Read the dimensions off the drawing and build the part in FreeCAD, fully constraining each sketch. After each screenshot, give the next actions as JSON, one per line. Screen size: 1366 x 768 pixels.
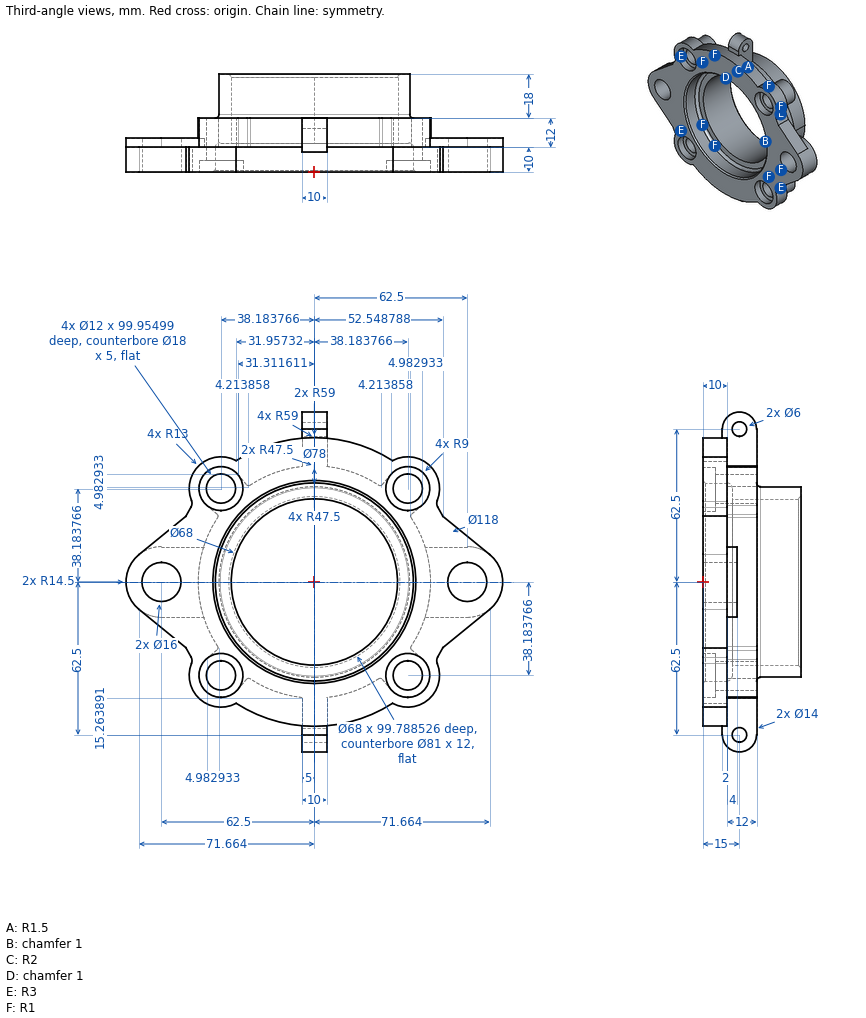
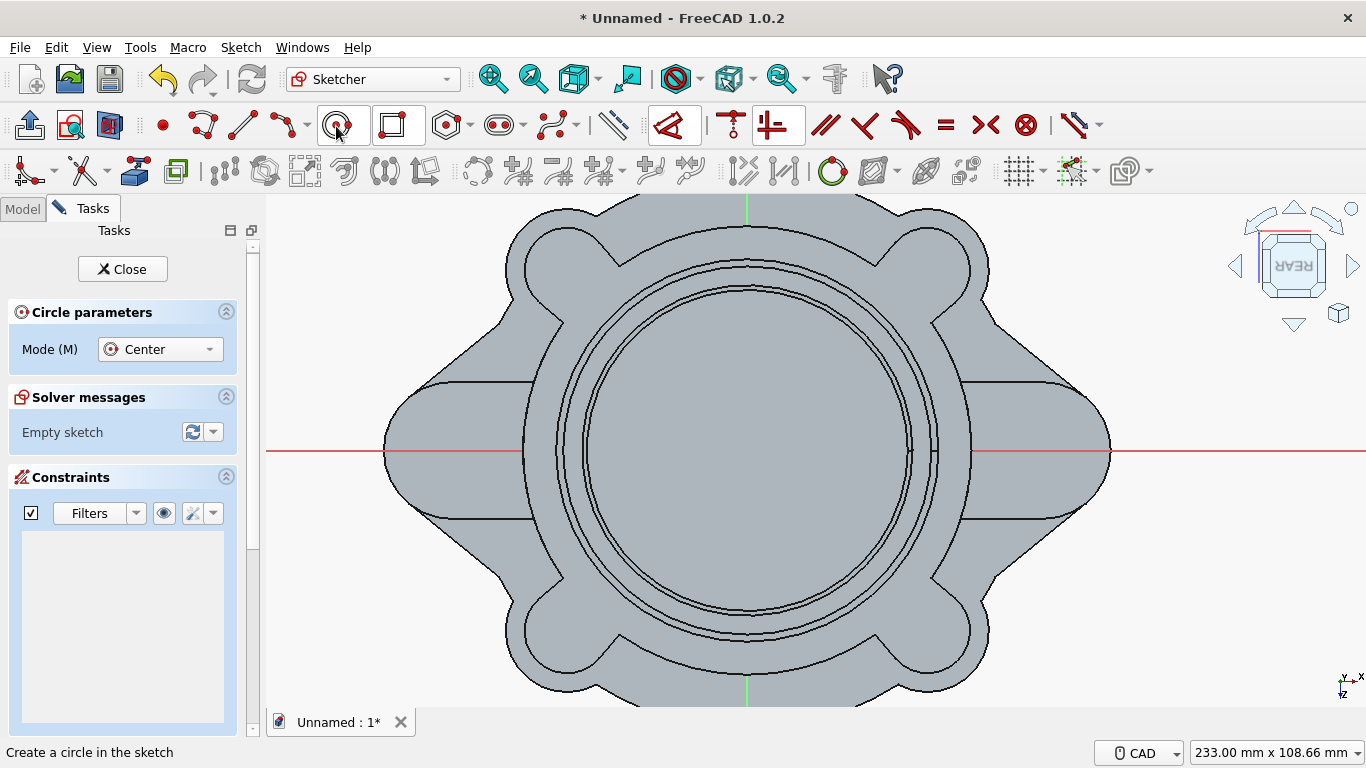
{"action": "left_click", "coordinate": [452, 450]}
{"action": "left_click", "coordinate": [479, 424]}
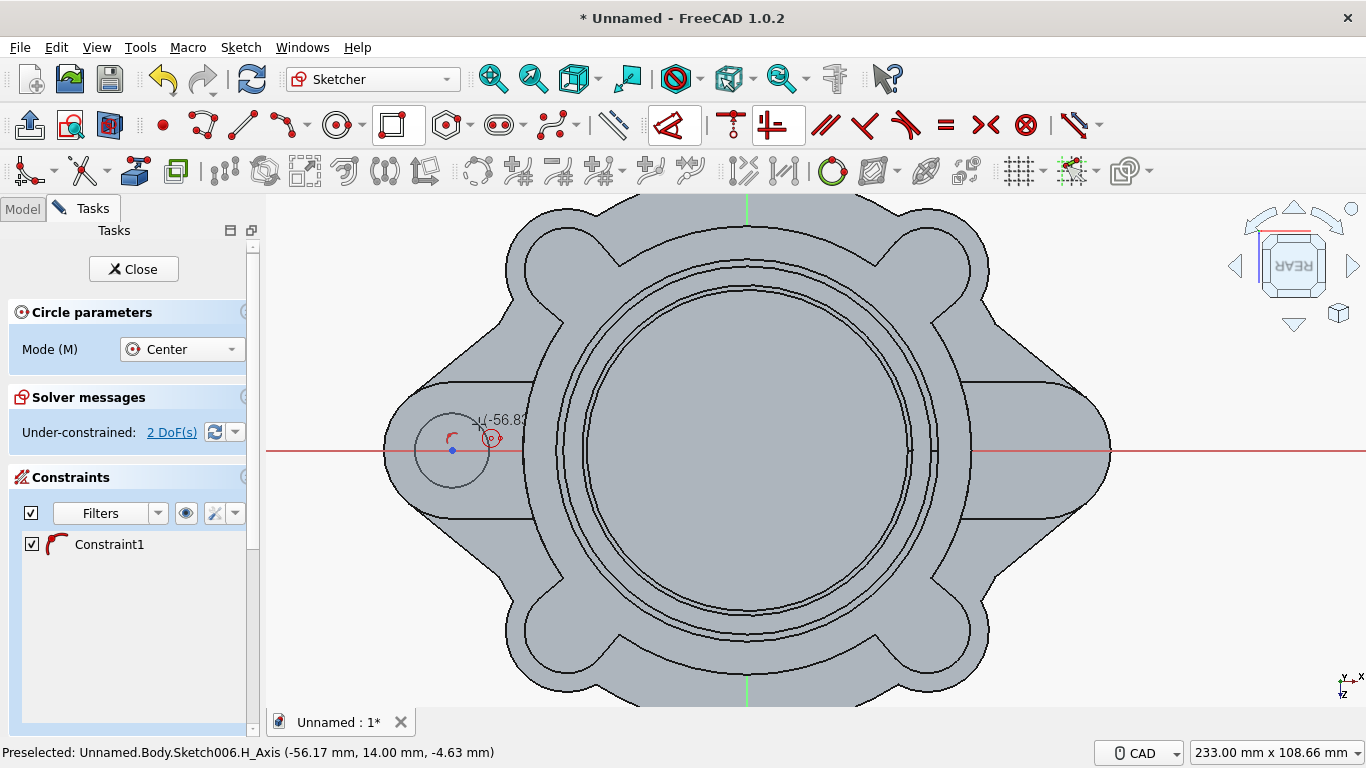
{"action": "left_click", "coordinate": [1042, 450]}
{"action": "left_click", "coordinate": [1069, 424]}
{"action": "key", "text": "Escape"}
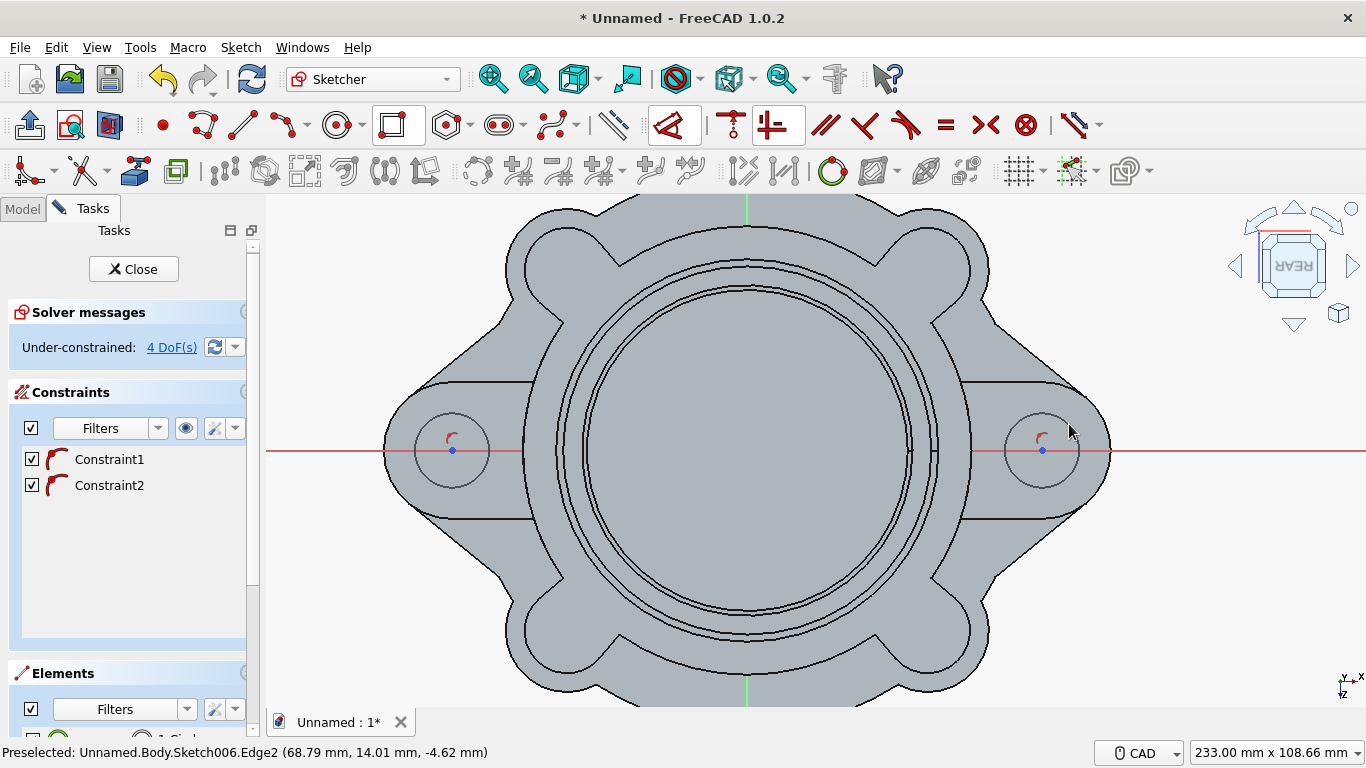
{"action": "left_click", "coordinate": [478, 424]}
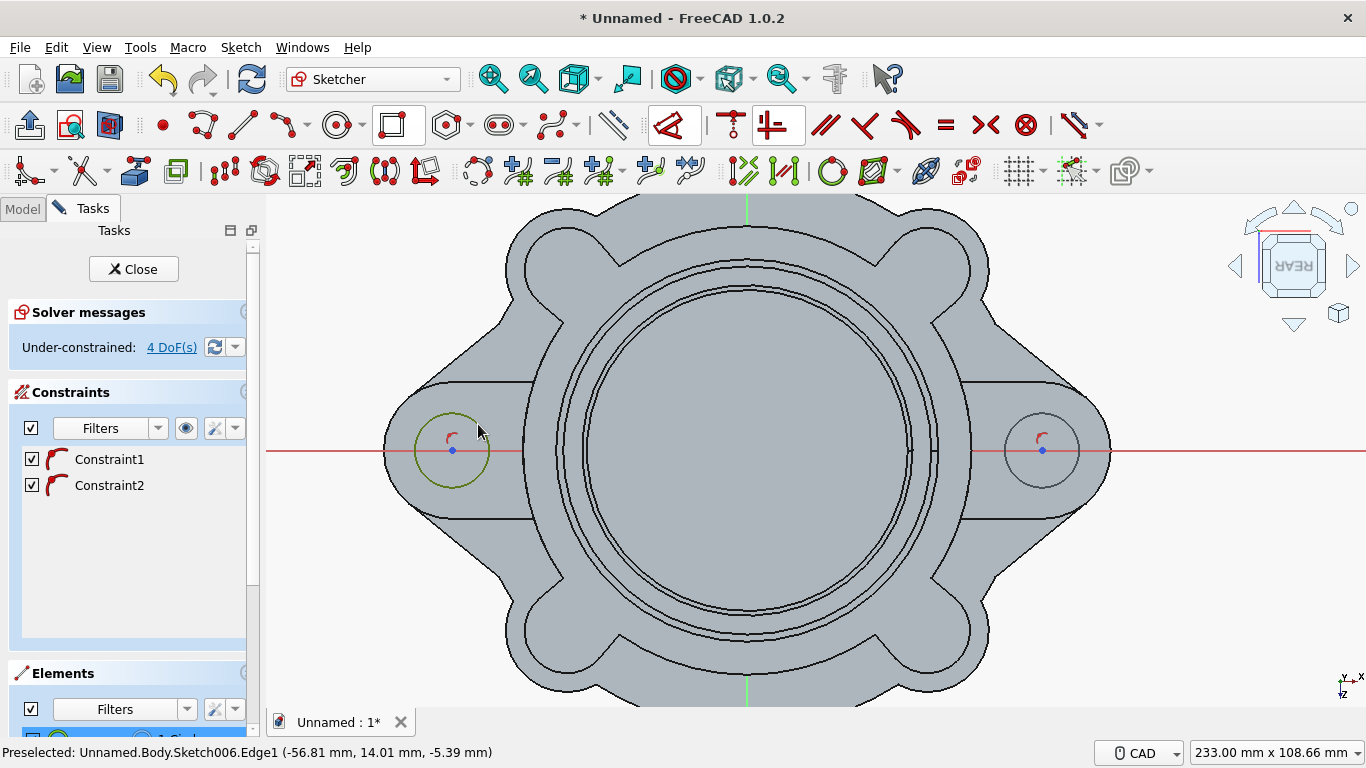
{"action": "left_click", "coordinate": [1068, 424]}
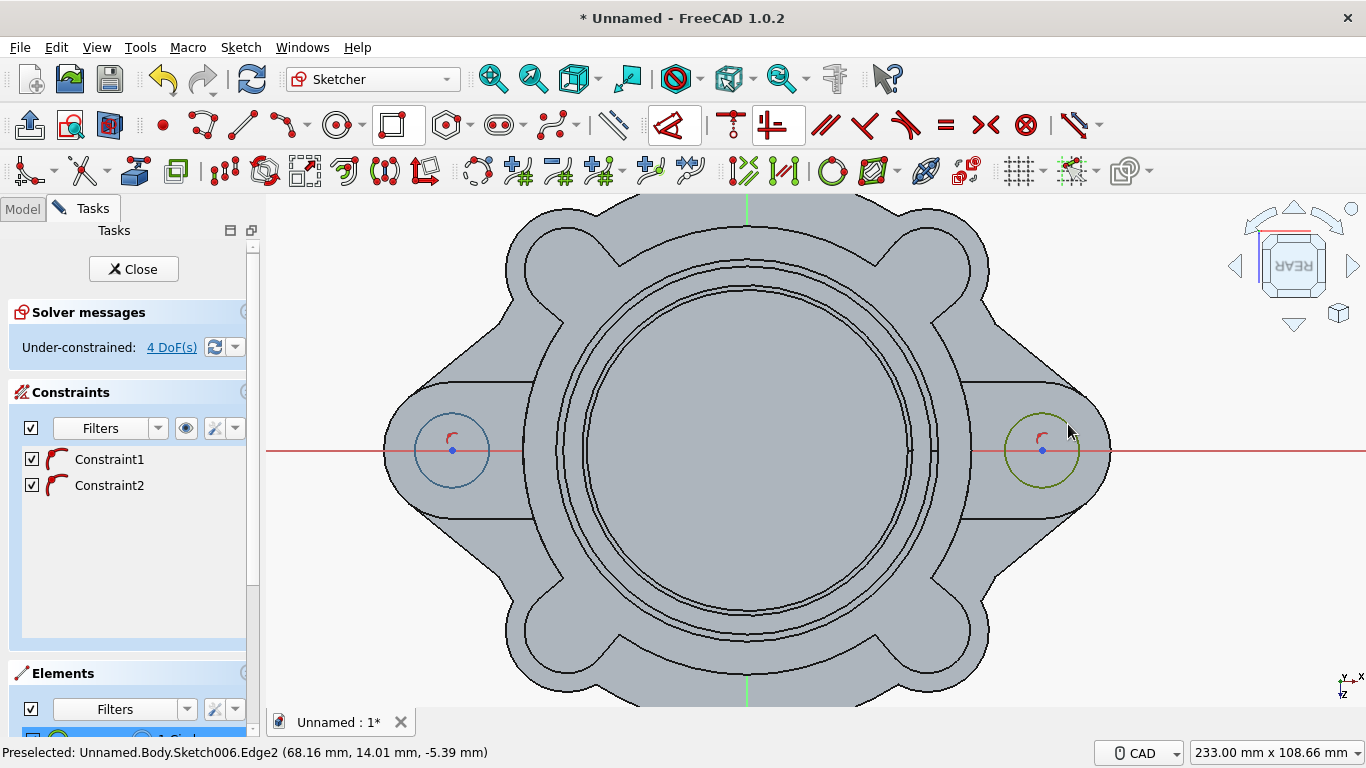
{"action": "left_click", "coordinate": [946, 126]}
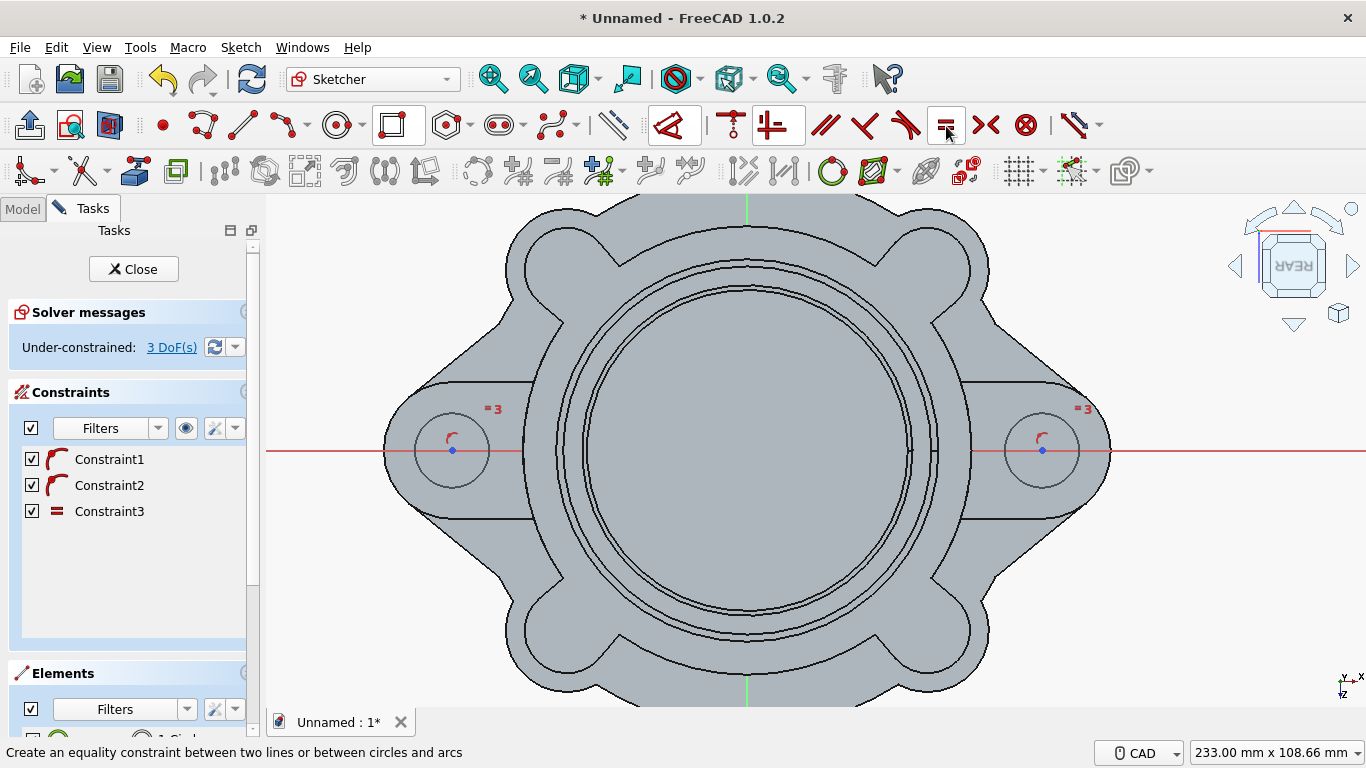
{"action": "left_click", "coordinate": [478, 424]}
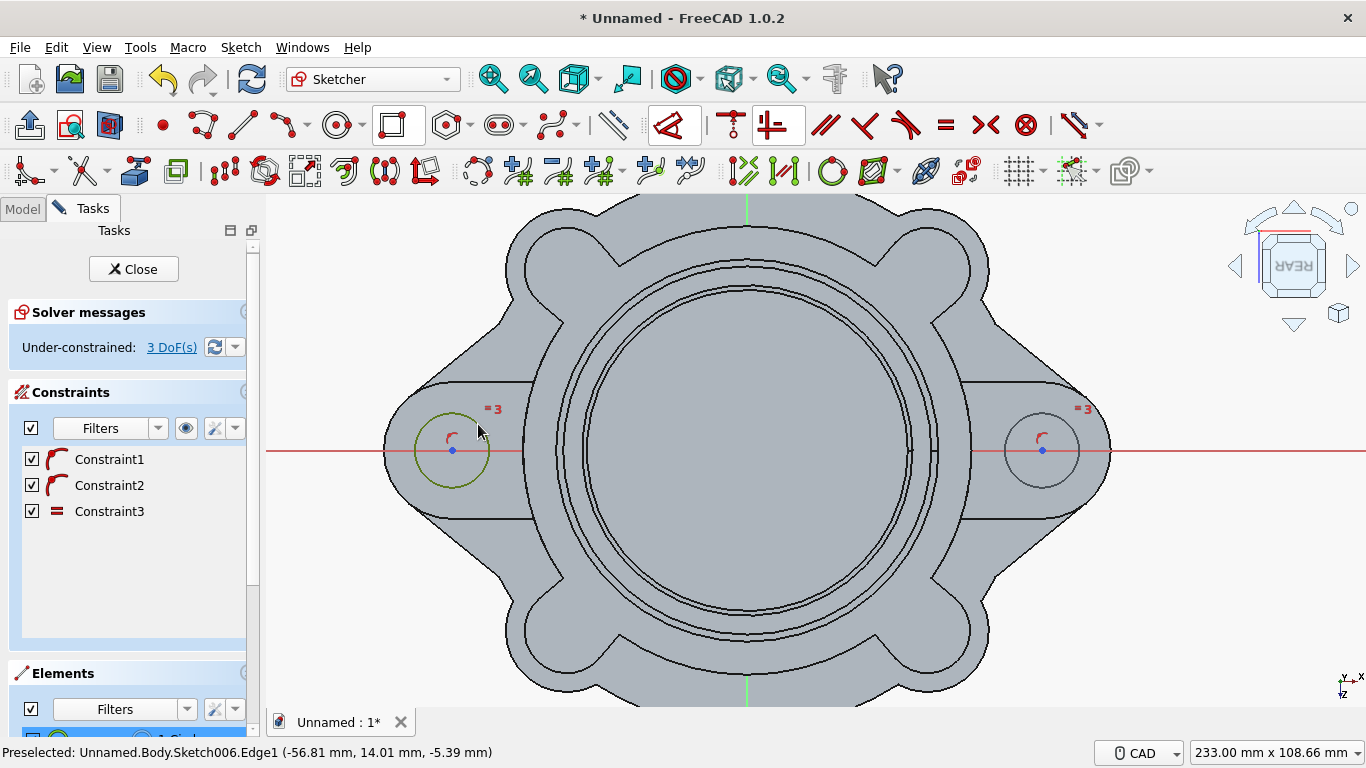
{"action": "left_click", "coordinate": [696, 126]}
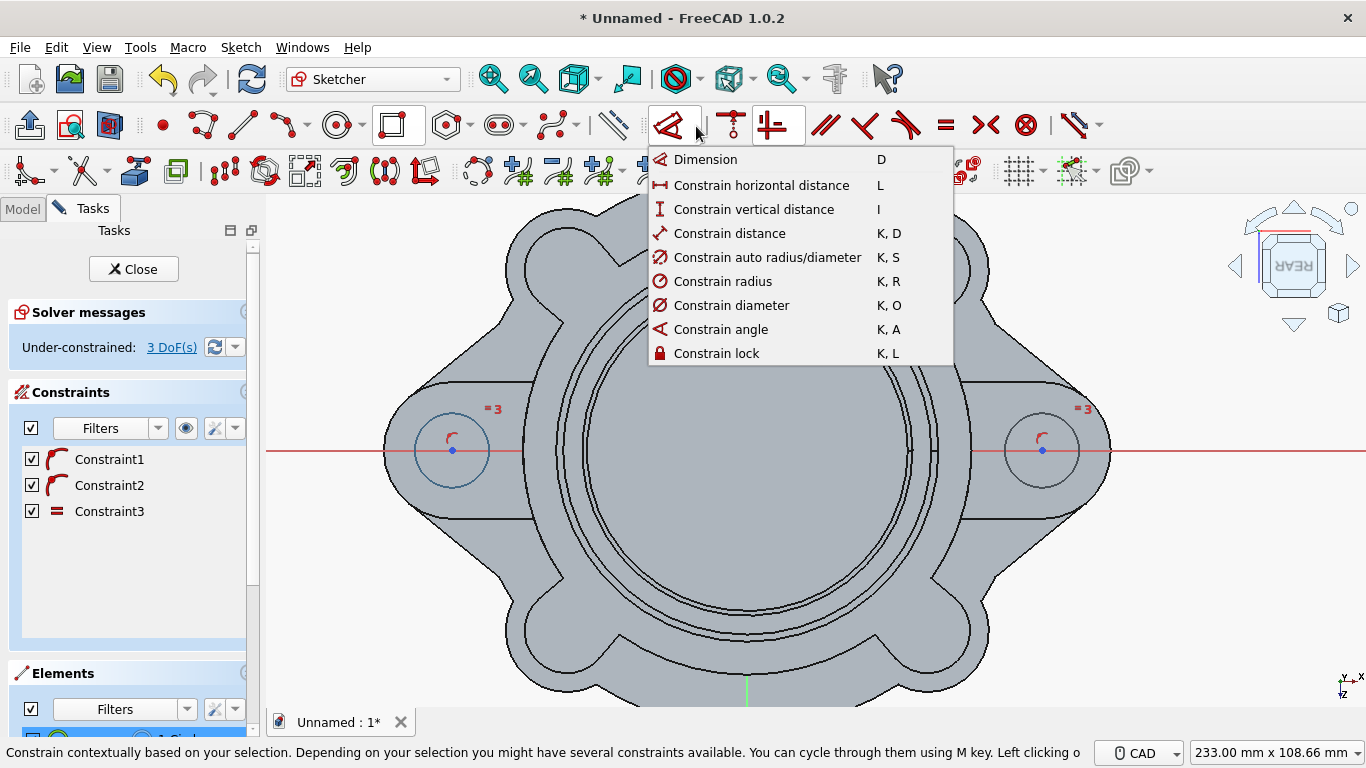
{"action": "left_click", "coordinate": [801, 305]}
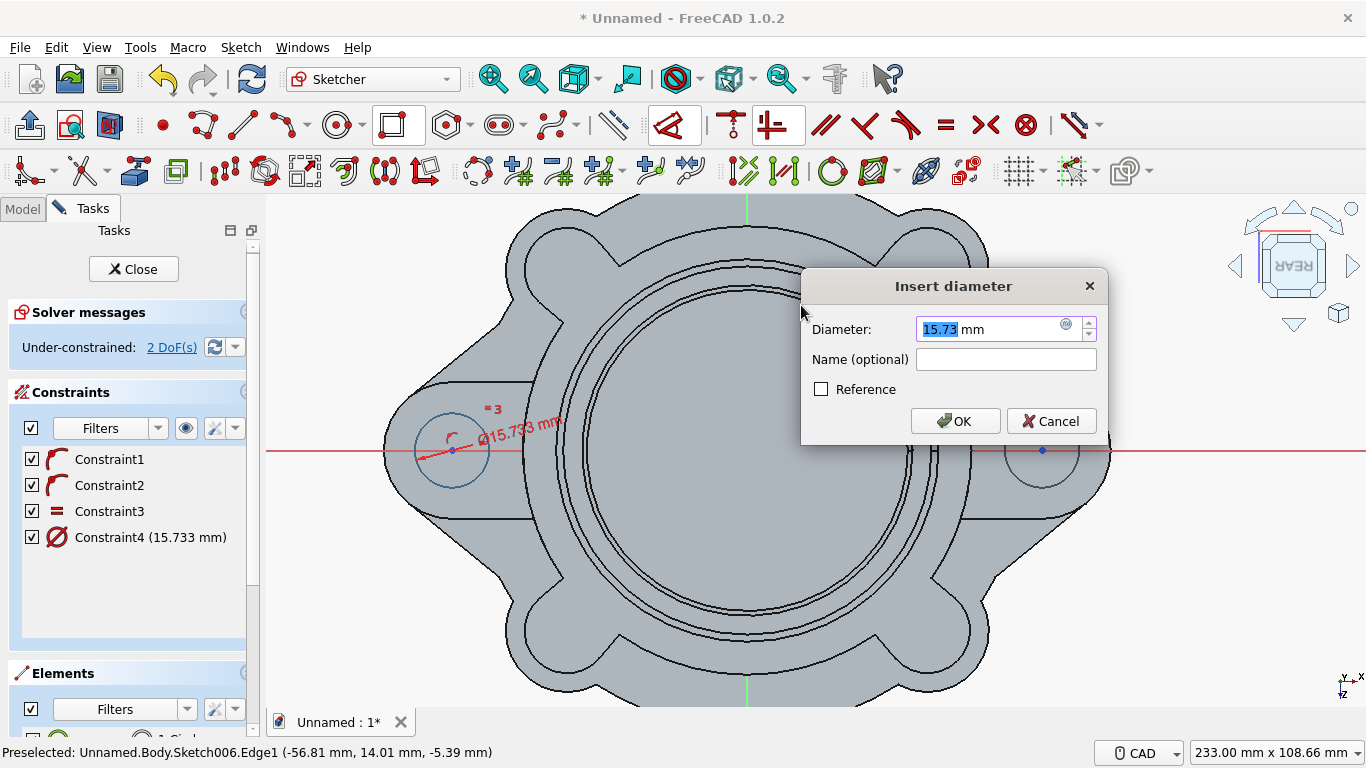
{"action": "type", "text": "16"}
{"action": "key", "text": "Return"}